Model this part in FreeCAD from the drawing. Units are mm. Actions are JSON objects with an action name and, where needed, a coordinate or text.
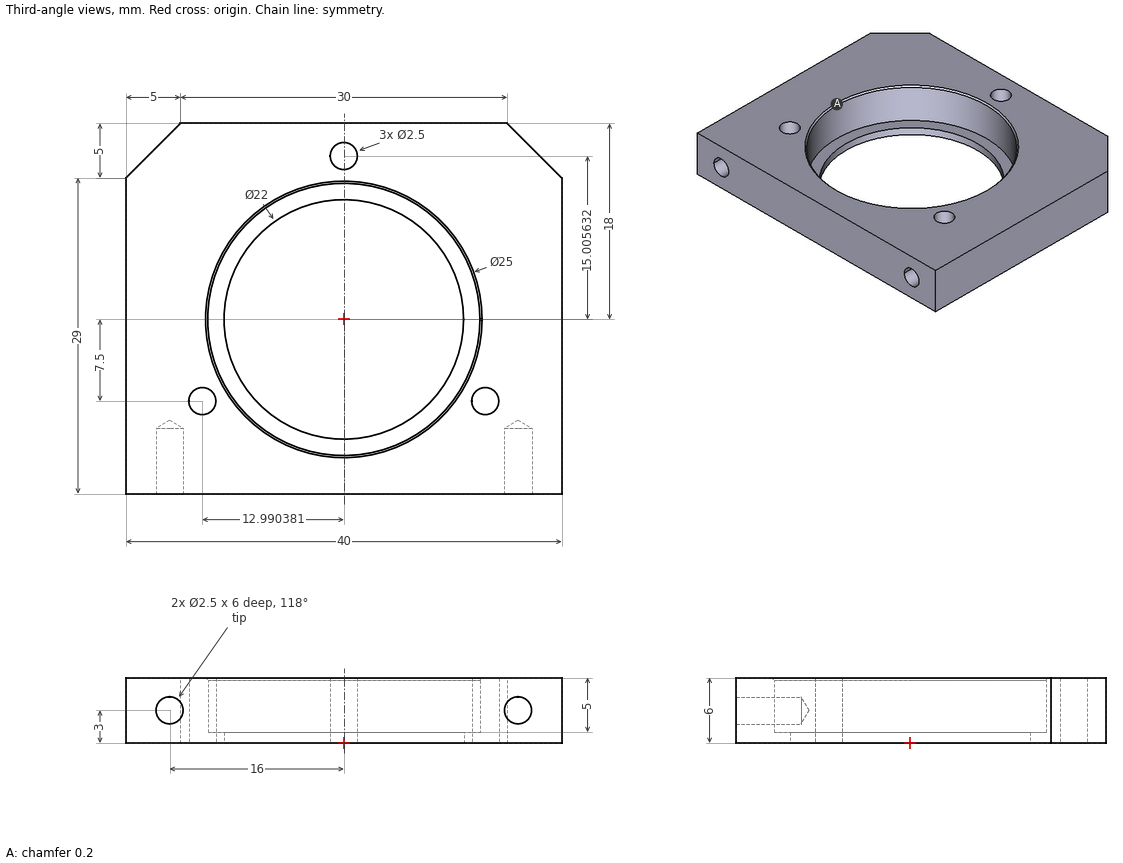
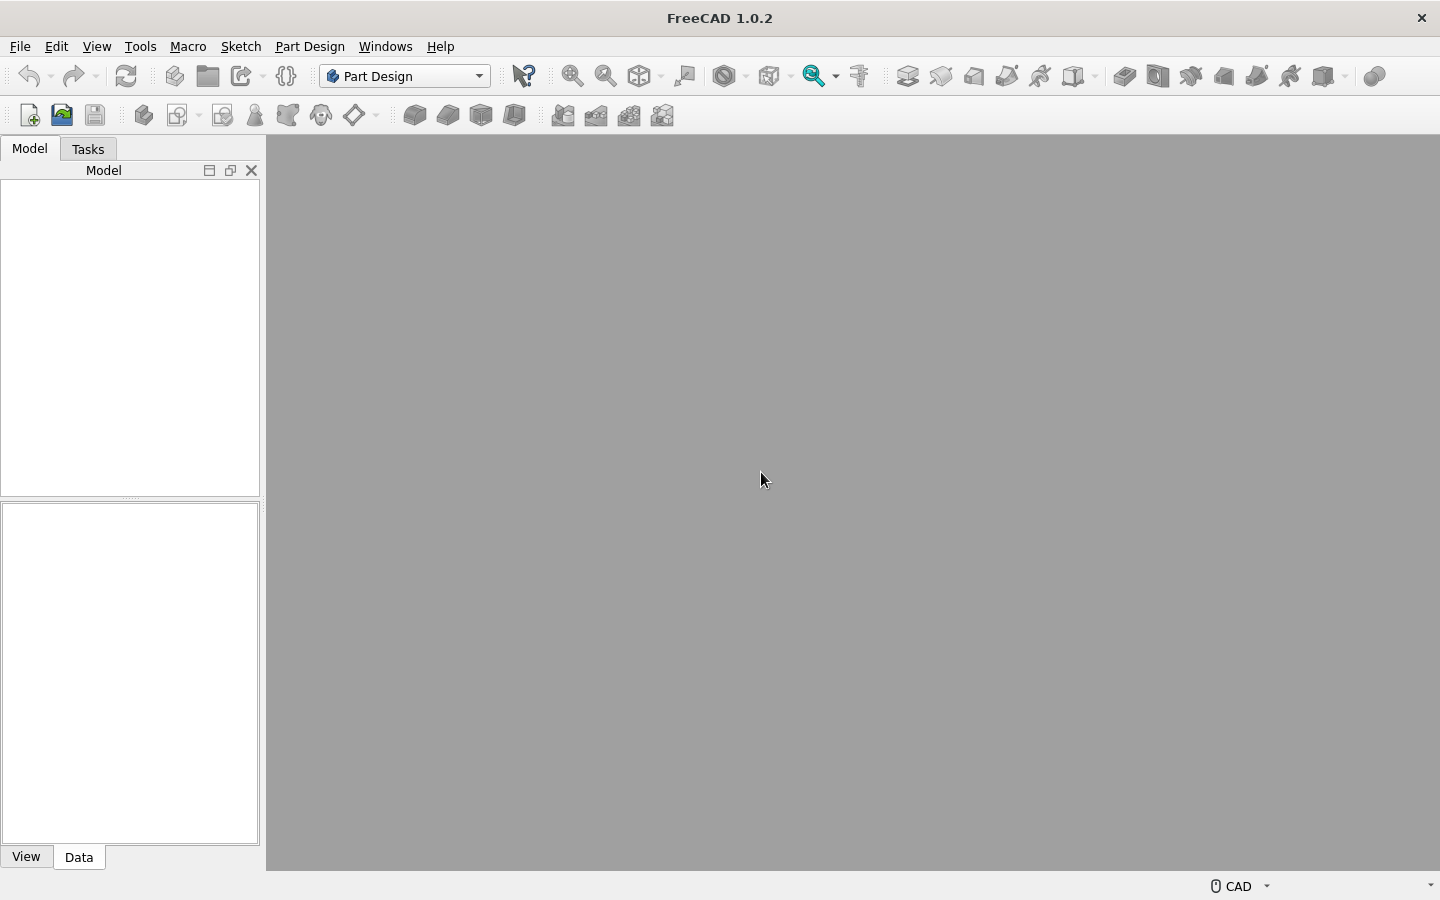
{"action": "left_click", "coordinate": [29, 116]}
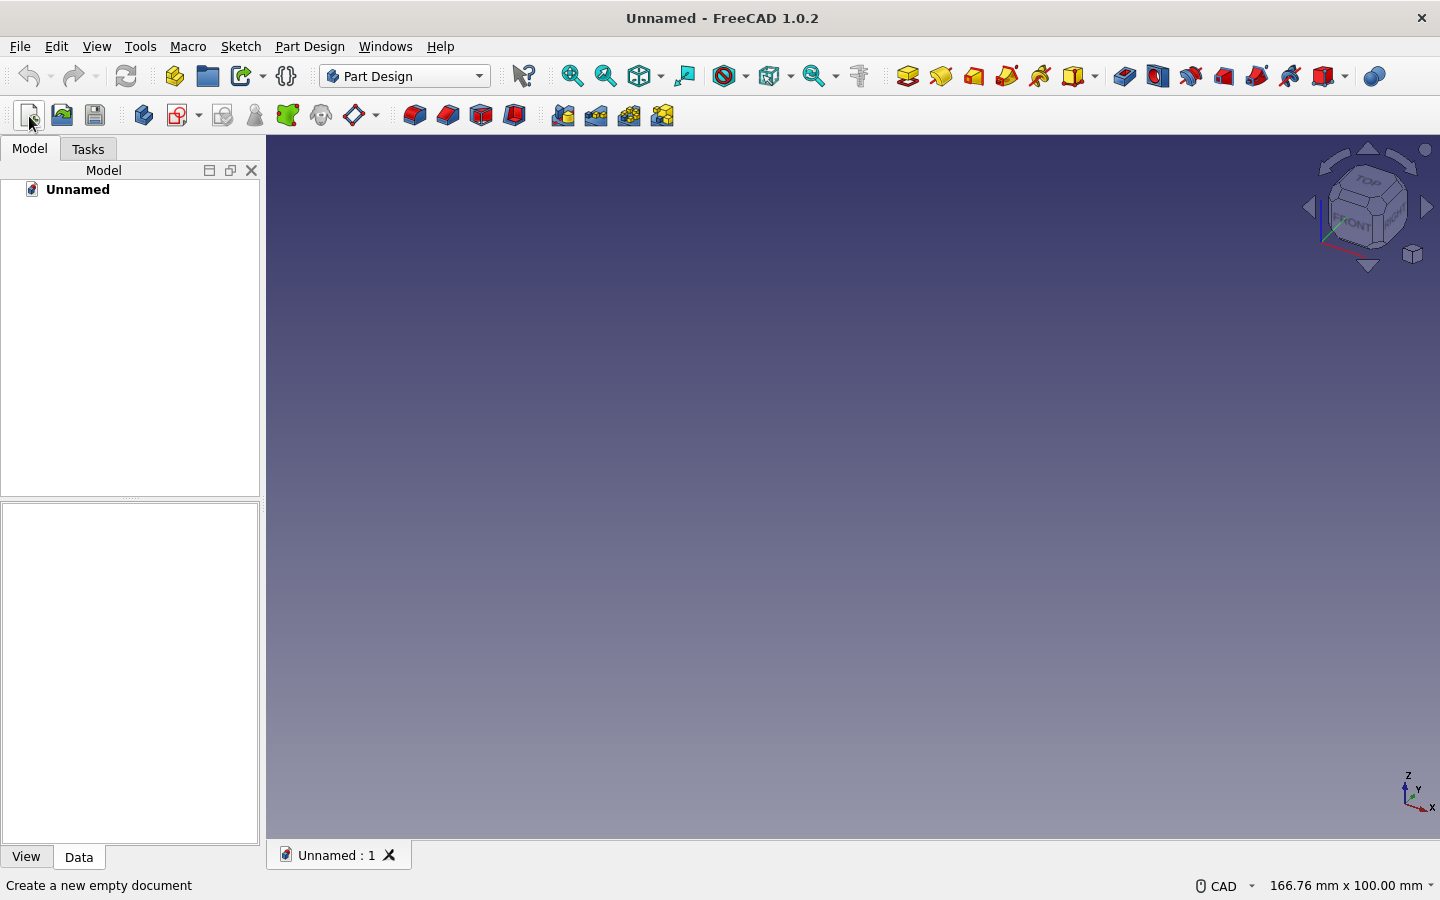
{"action": "left_click", "coordinate": [176, 116]}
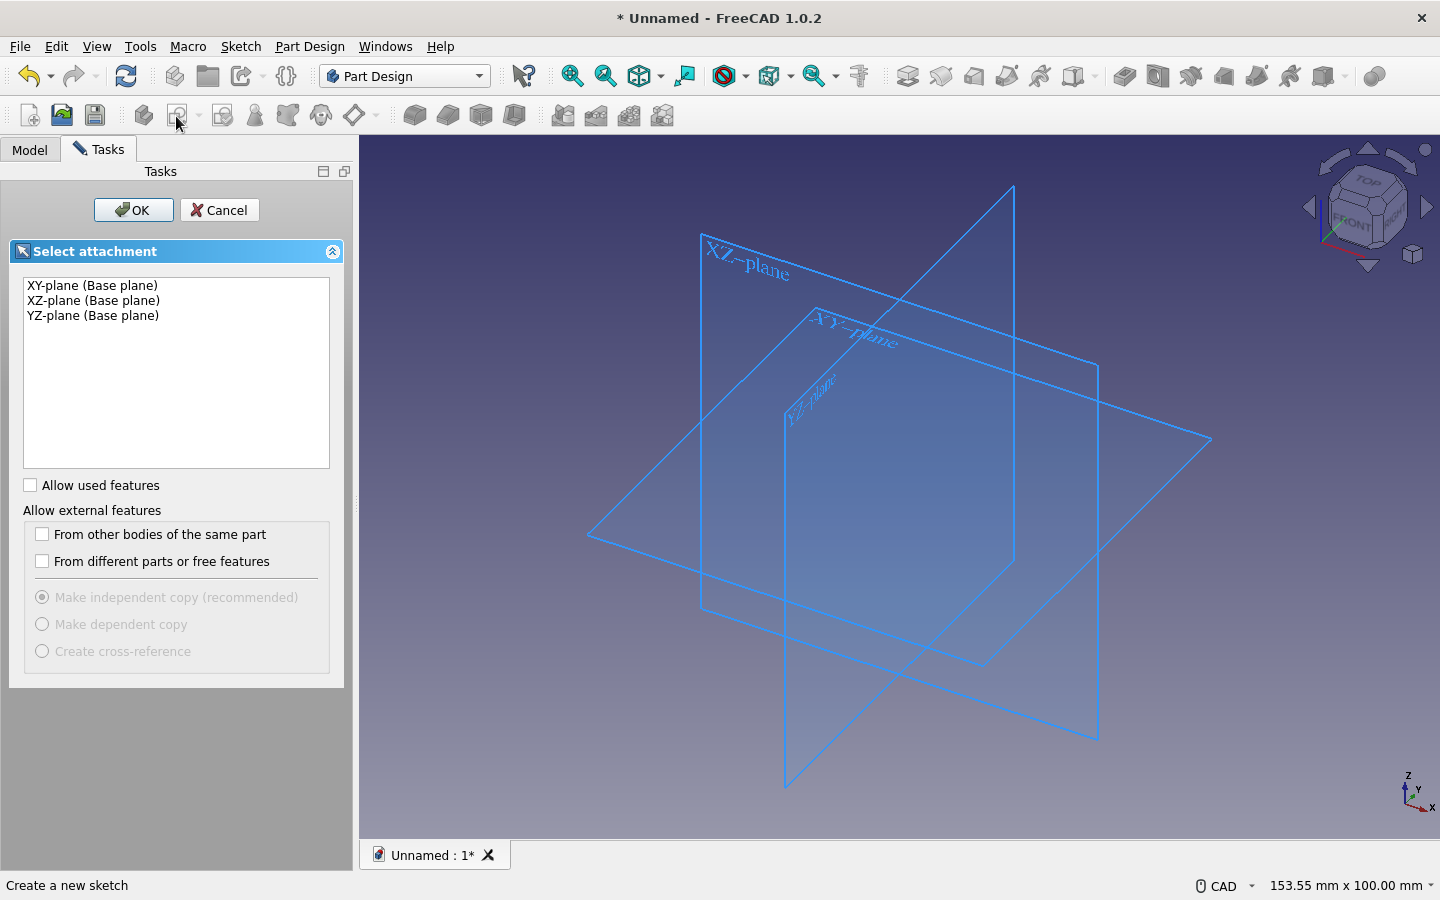
{"action": "left_click", "coordinate": [84, 286]}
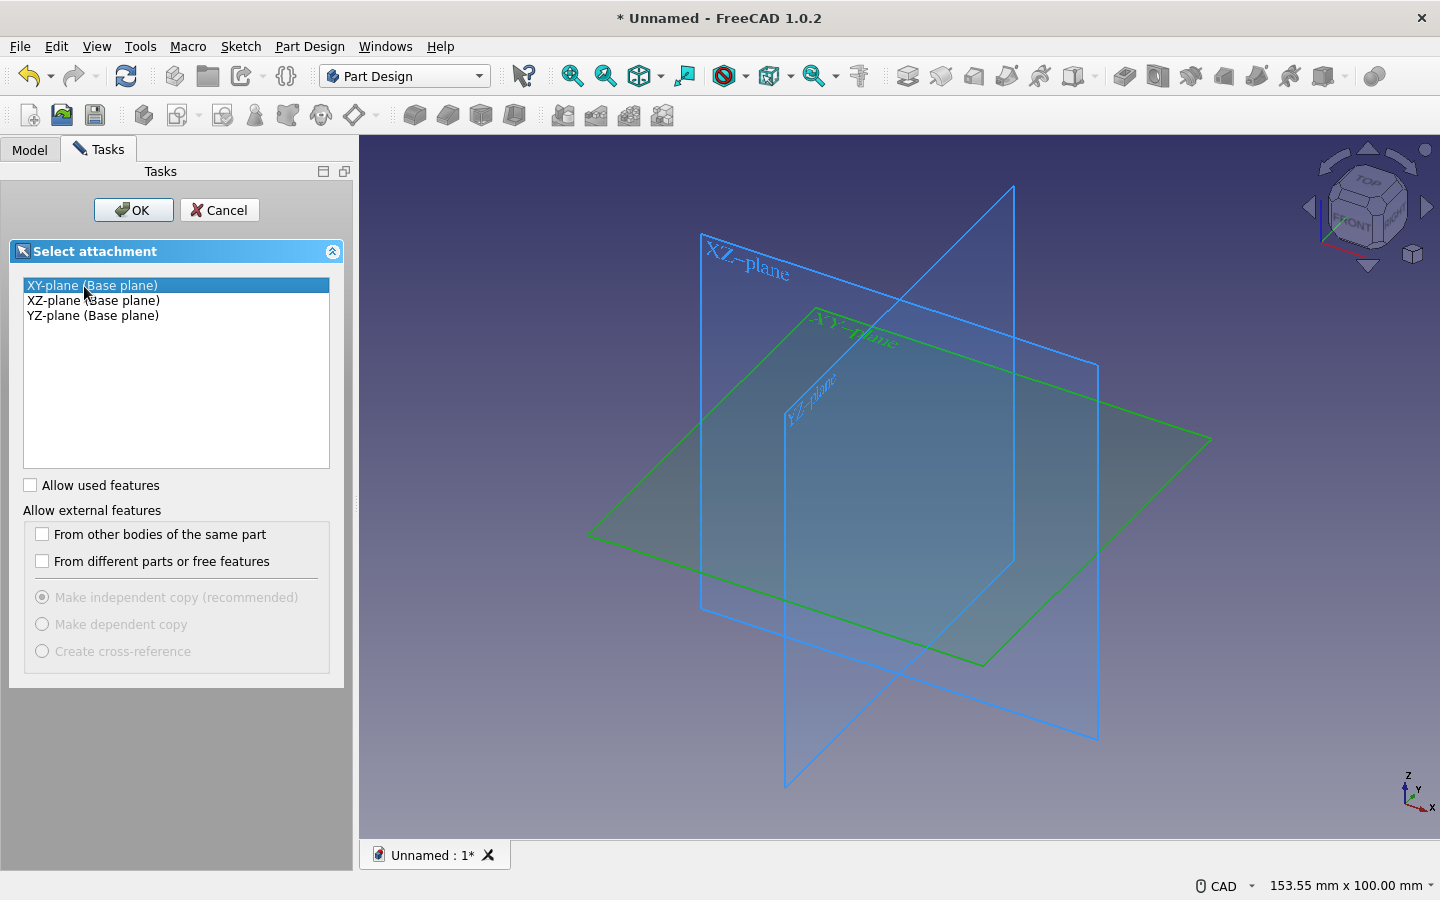
{"action": "left_click", "coordinate": [134, 210]}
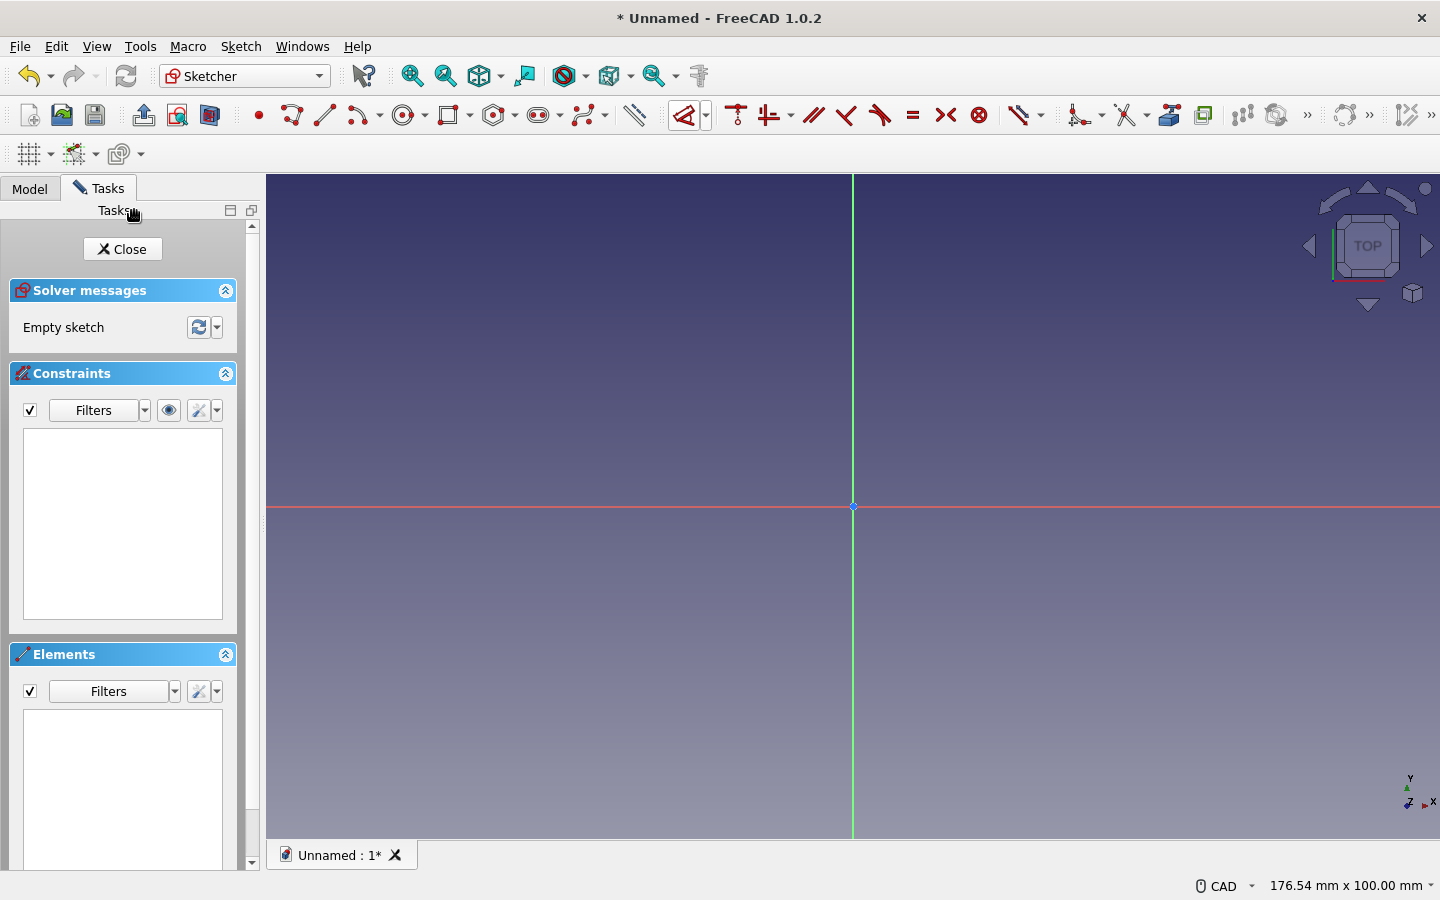
{"action": "scroll", "coordinate": [936, 492], "scroll_direction": "up", "scroll_amount": 3}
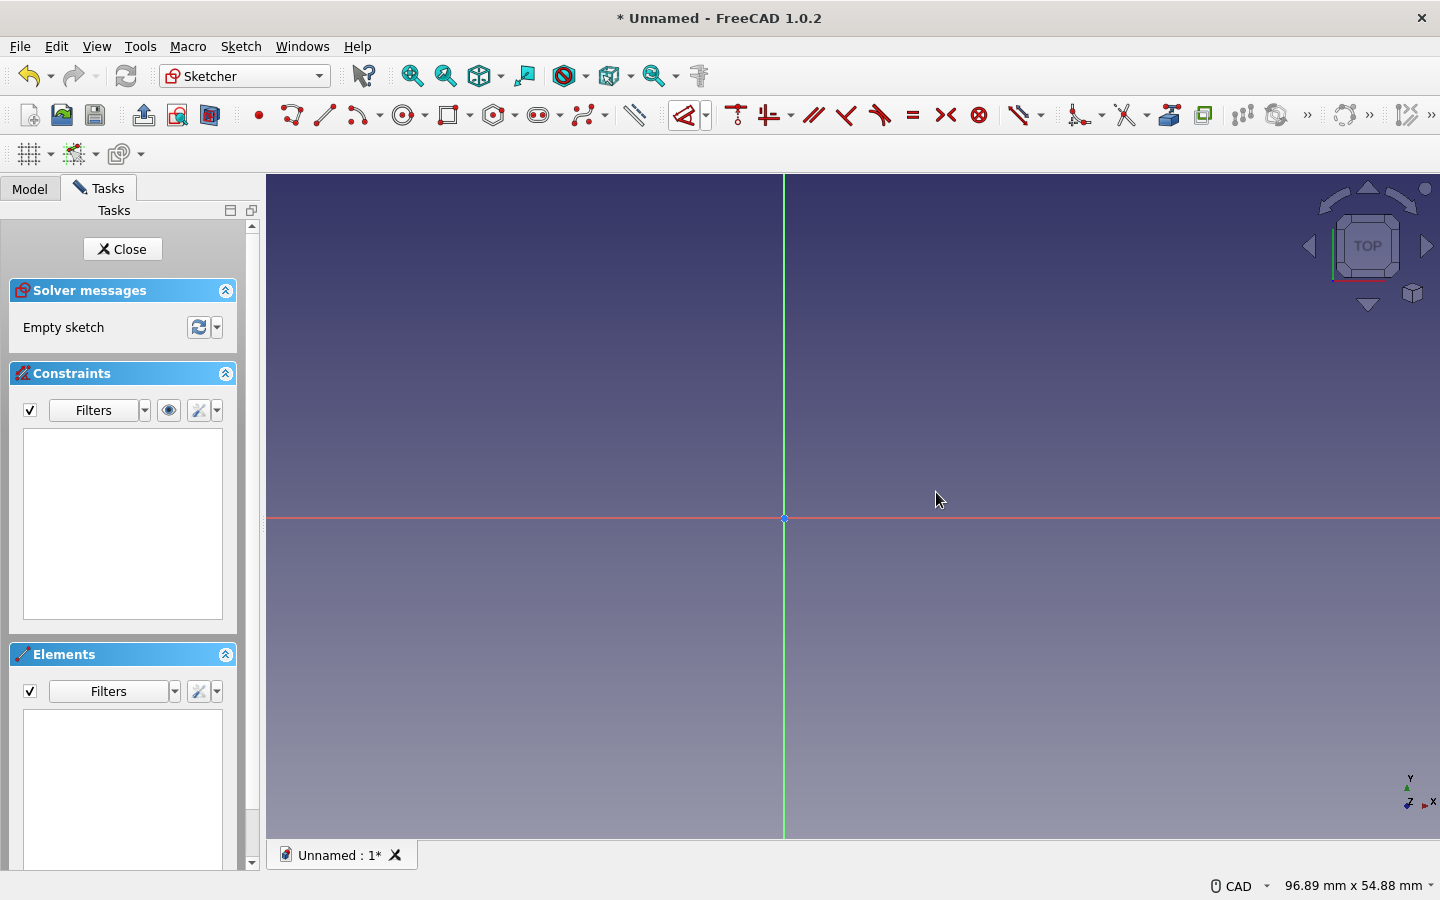
{"action": "left_click", "coordinate": [292, 116]}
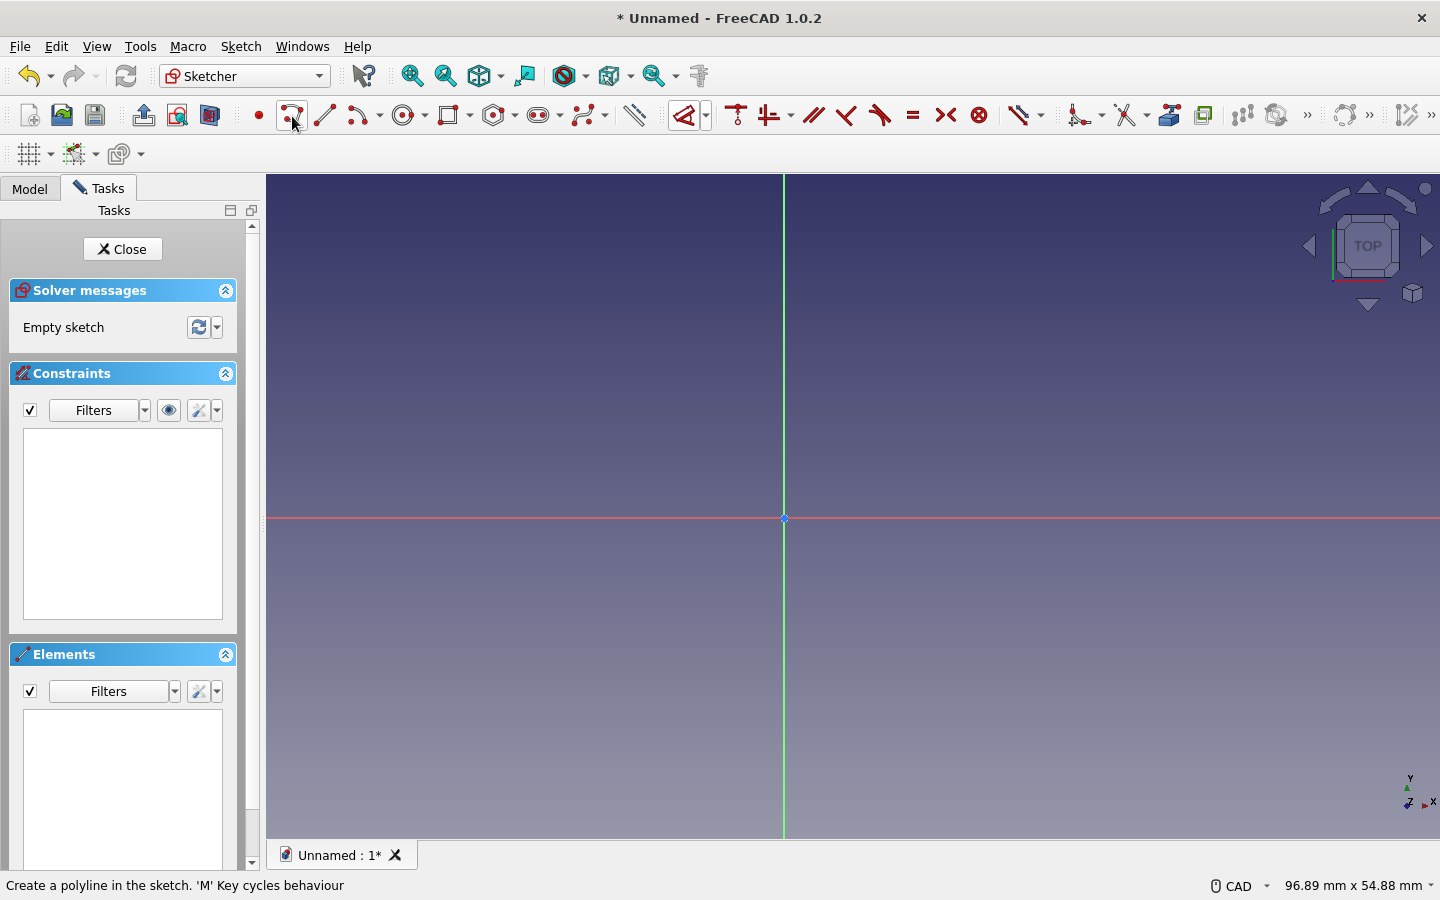
{"action": "left_click", "coordinate": [966, 300]}
{"action": "left_click", "coordinate": [603, 300]}
{"action": "left_click", "coordinate": [542, 361]}
{"action": "left_click", "coordinate": [542, 712]}
{"action": "left_click", "coordinate": [1027, 712]}
{"action": "left_click", "coordinate": [1027, 361]}
{"action": "left_click", "coordinate": [966, 301]}